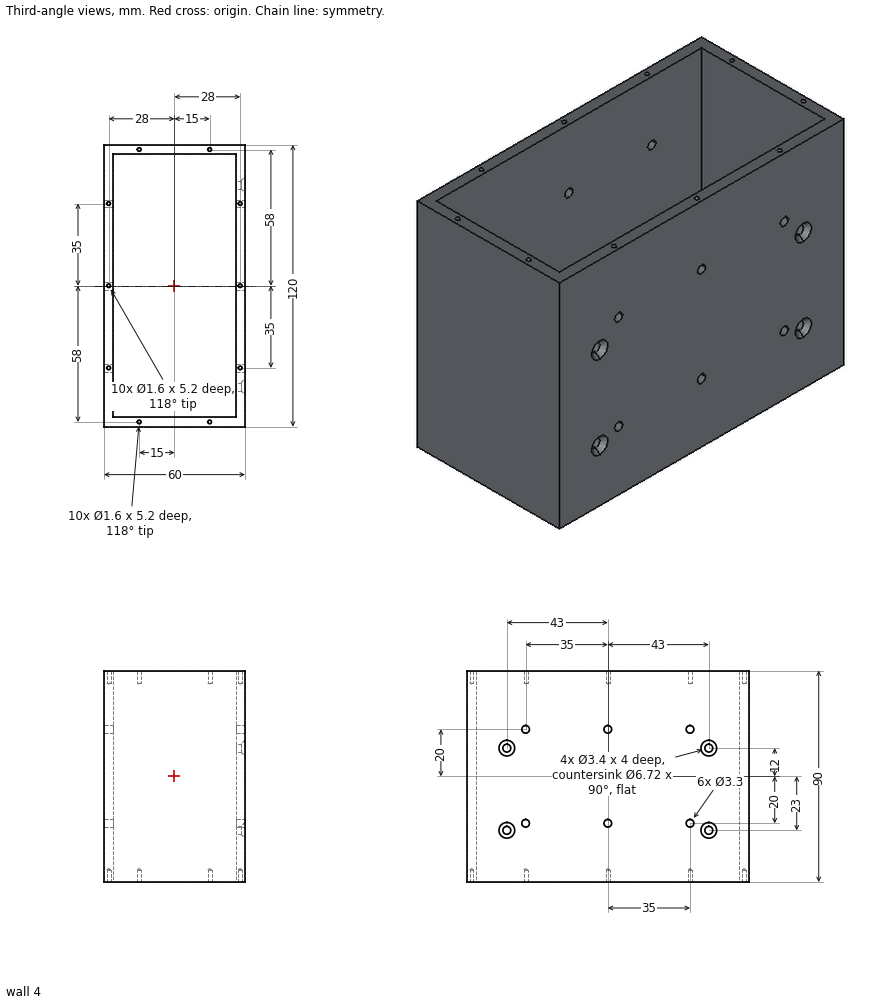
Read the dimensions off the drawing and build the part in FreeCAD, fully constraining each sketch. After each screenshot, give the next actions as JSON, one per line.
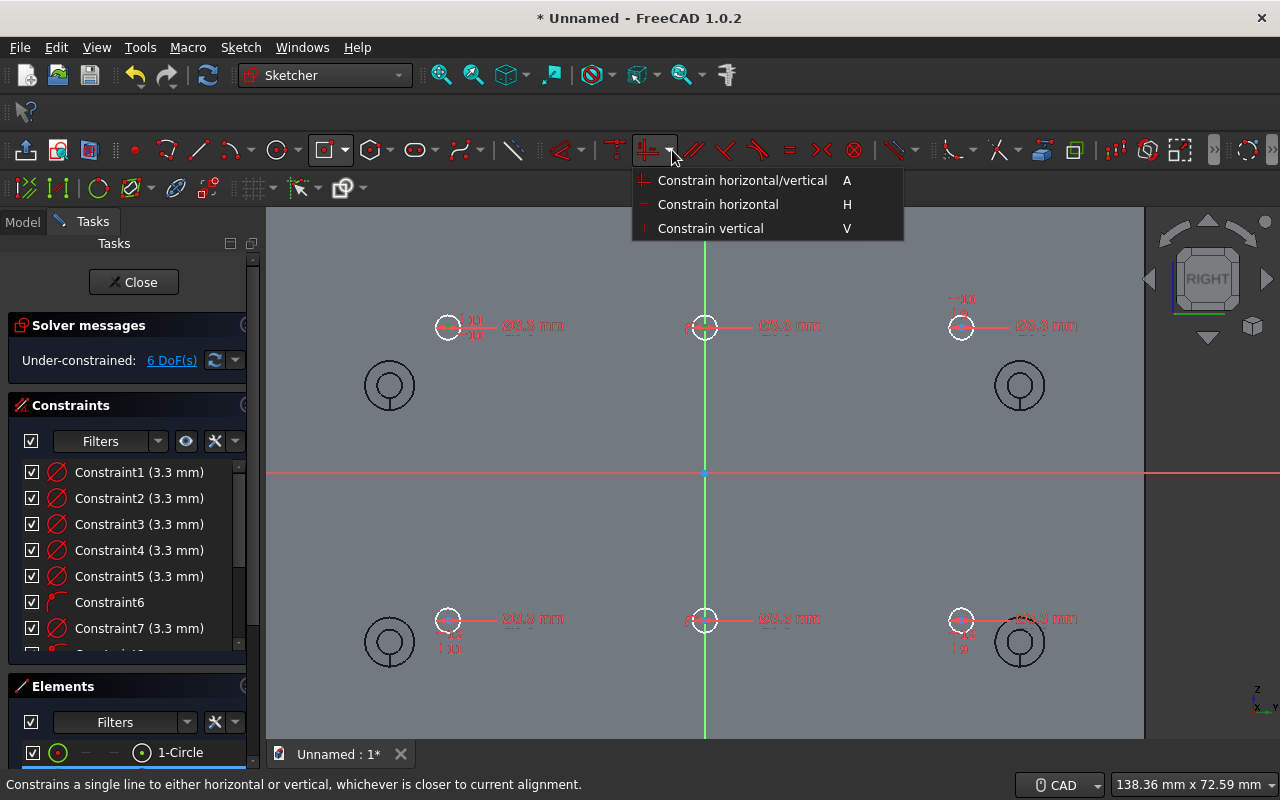
{"action": "left_click", "coordinate": [768, 204]}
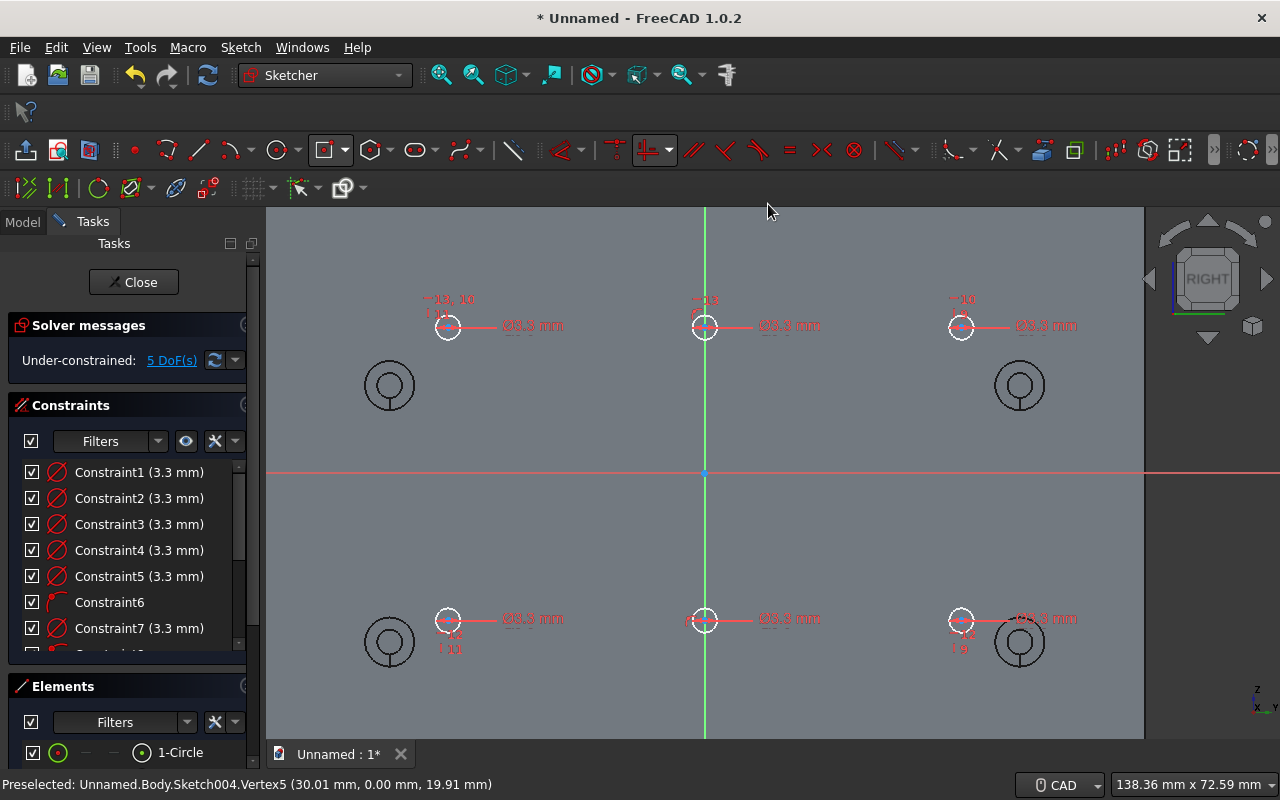
{"action": "left_click", "coordinate": [961, 621]}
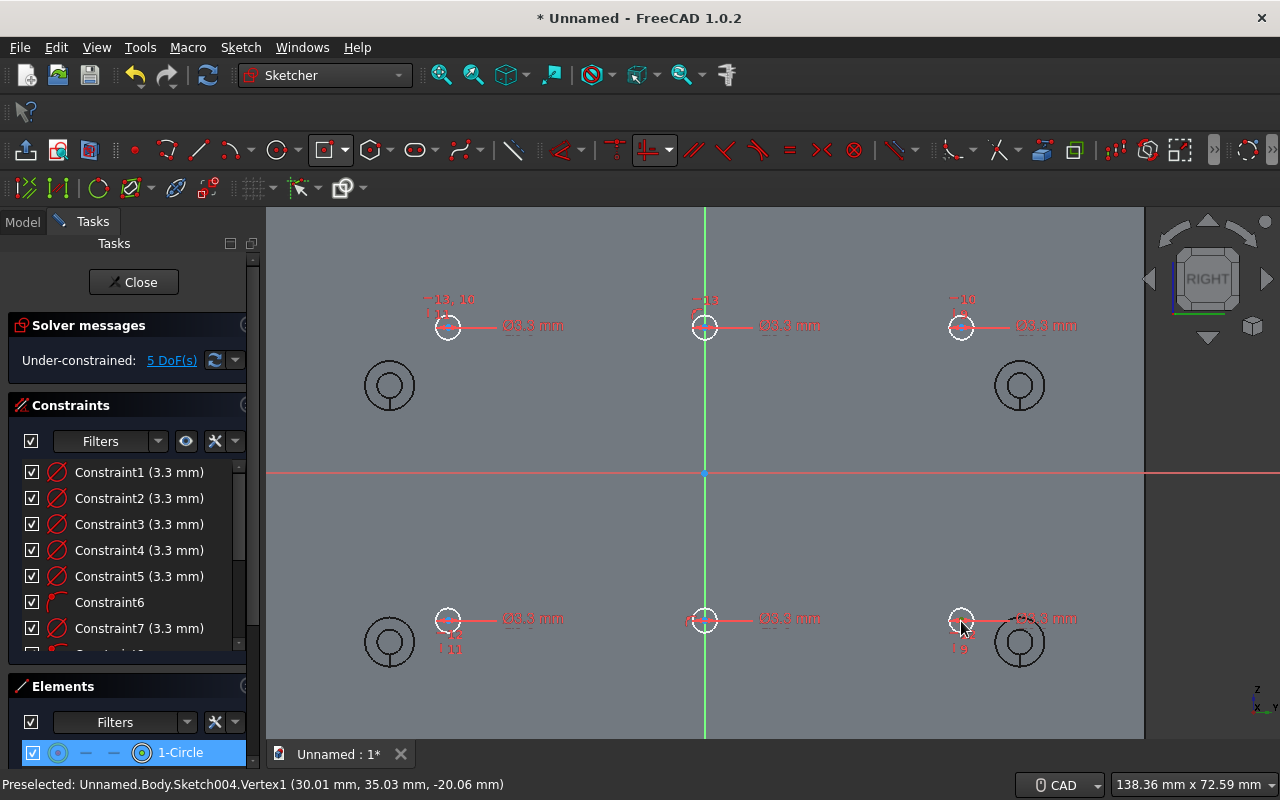
{"action": "left_click", "coordinate": [705, 621]}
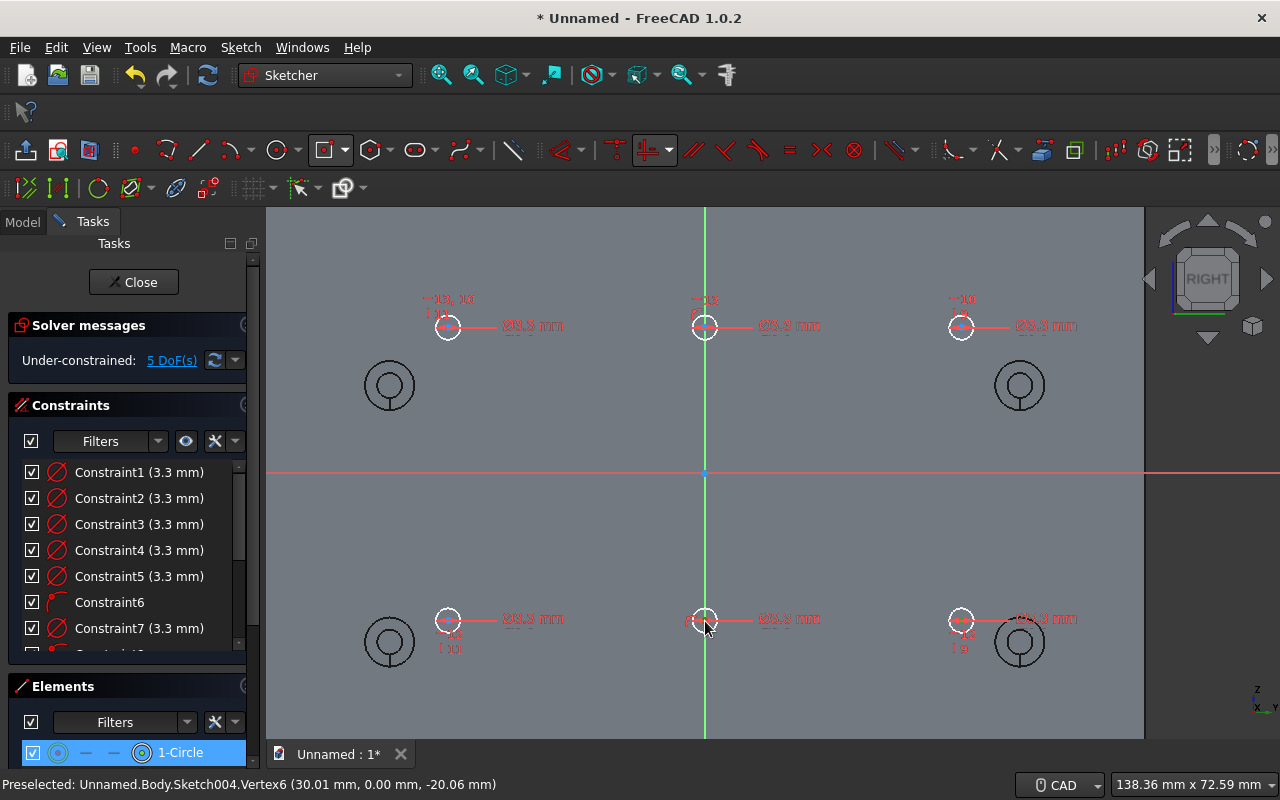
{"action": "left_click", "coordinate": [672, 150]}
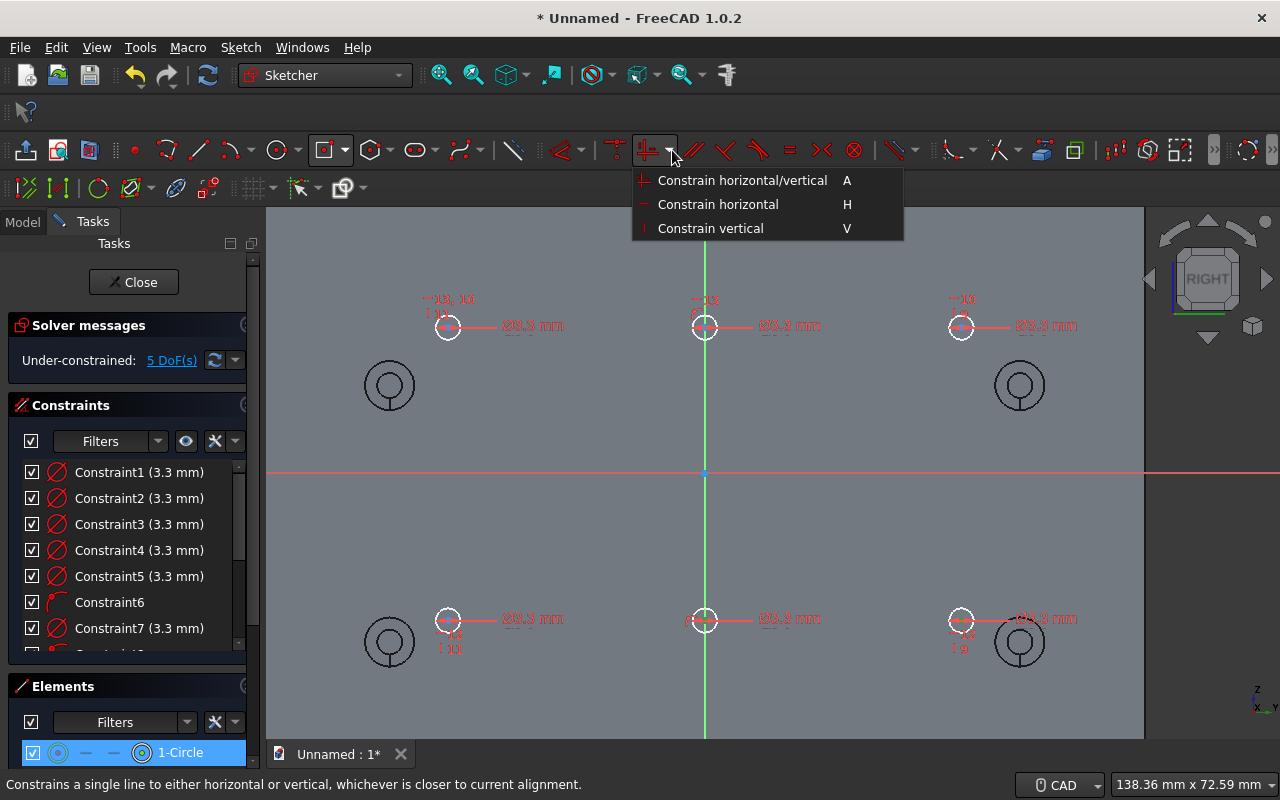
{"action": "left_click", "coordinate": [768, 204]}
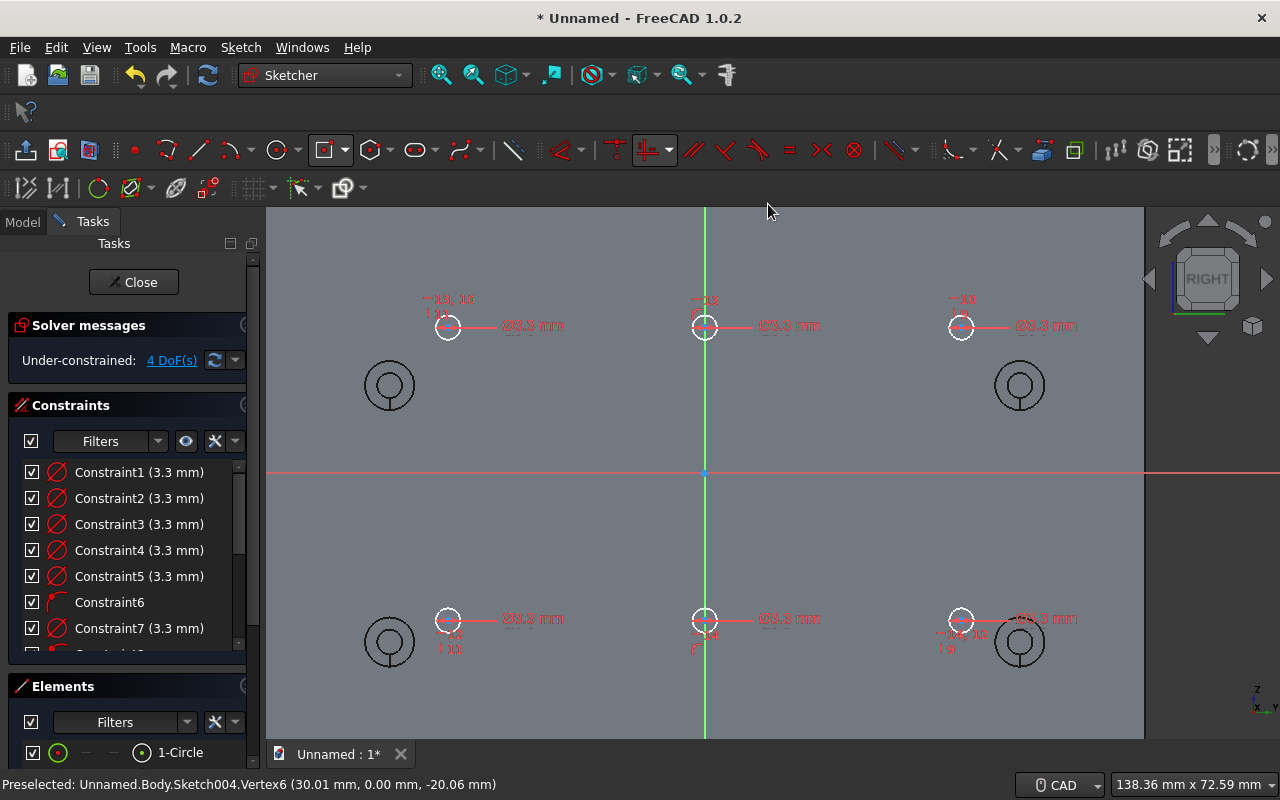
{"action": "left_click", "coordinate": [560, 150]}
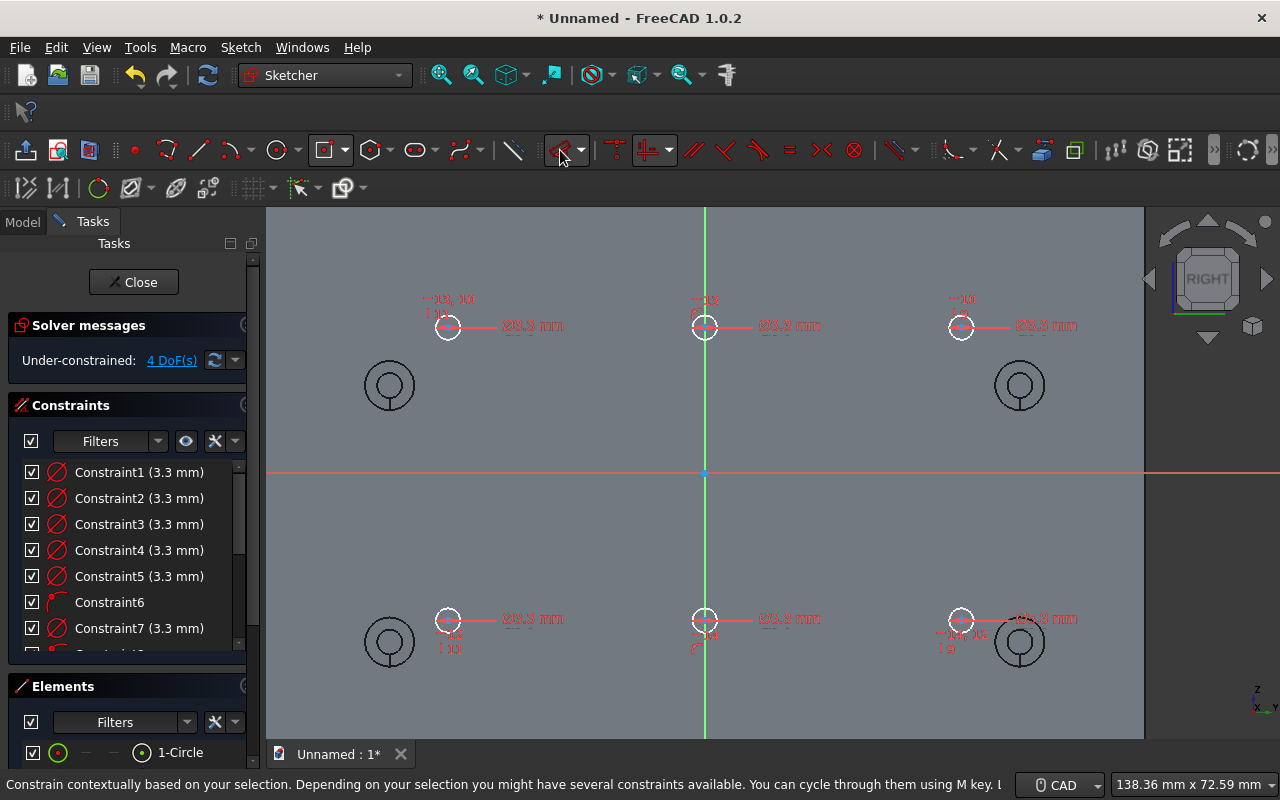
{"action": "left_click", "coordinate": [961, 621]}
{"action": "left_click", "coordinate": [833, 655]}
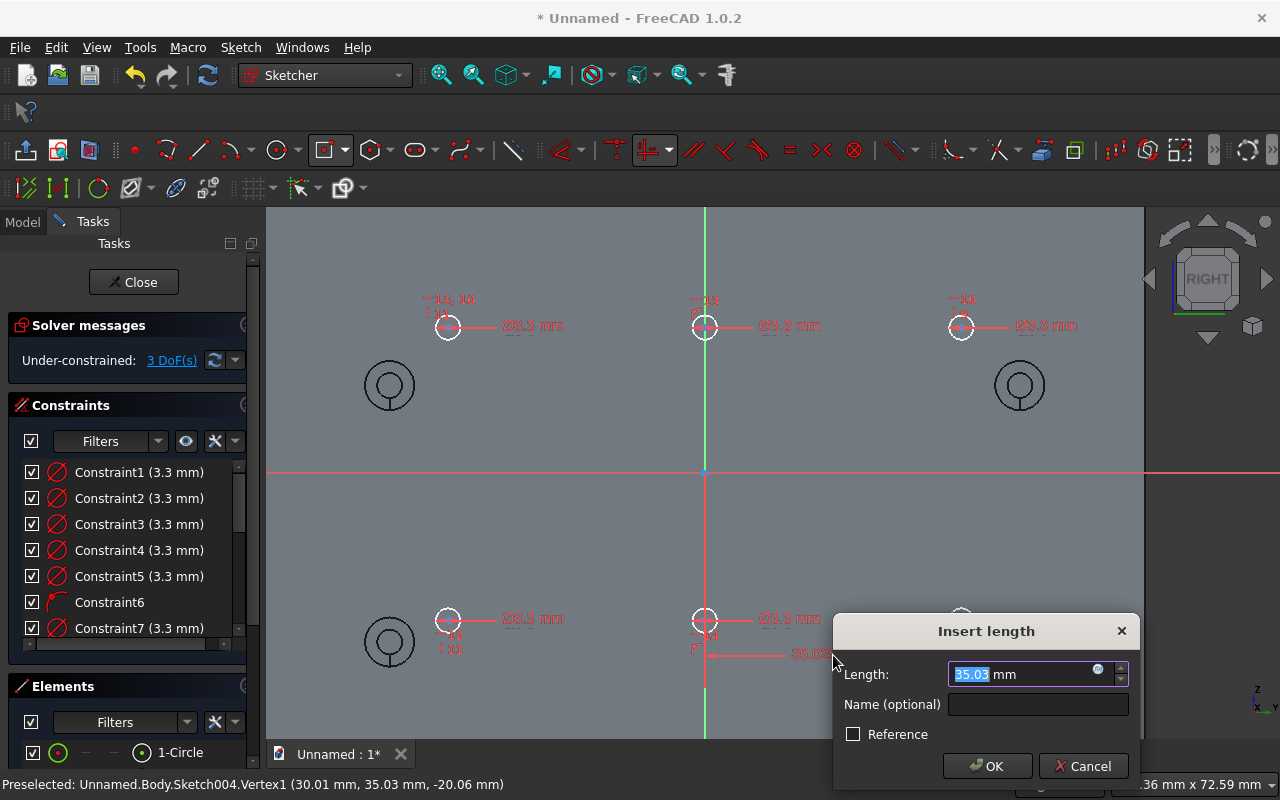
{"action": "type", "text": "35"}
{"action": "key", "text": "Return"}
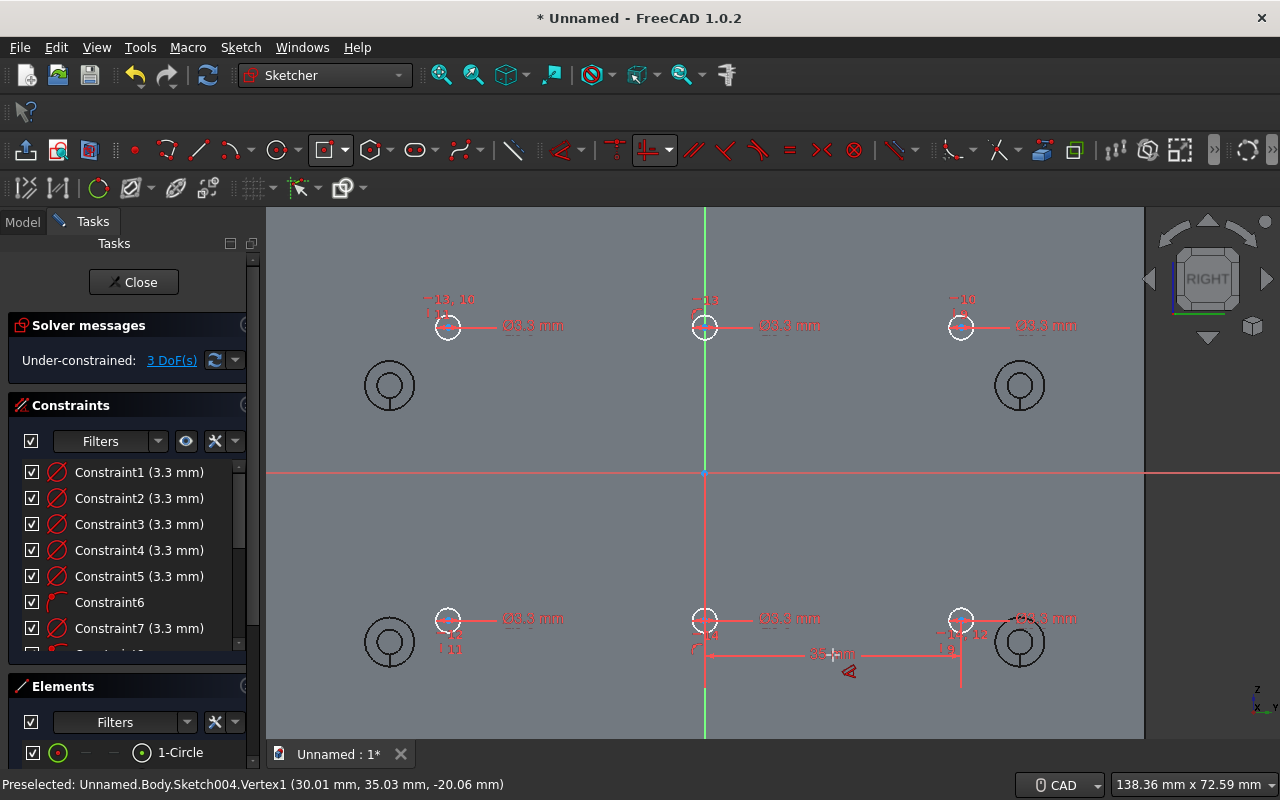
{"action": "left_click", "coordinate": [961, 621]}
{"action": "left_click", "coordinate": [995, 547]}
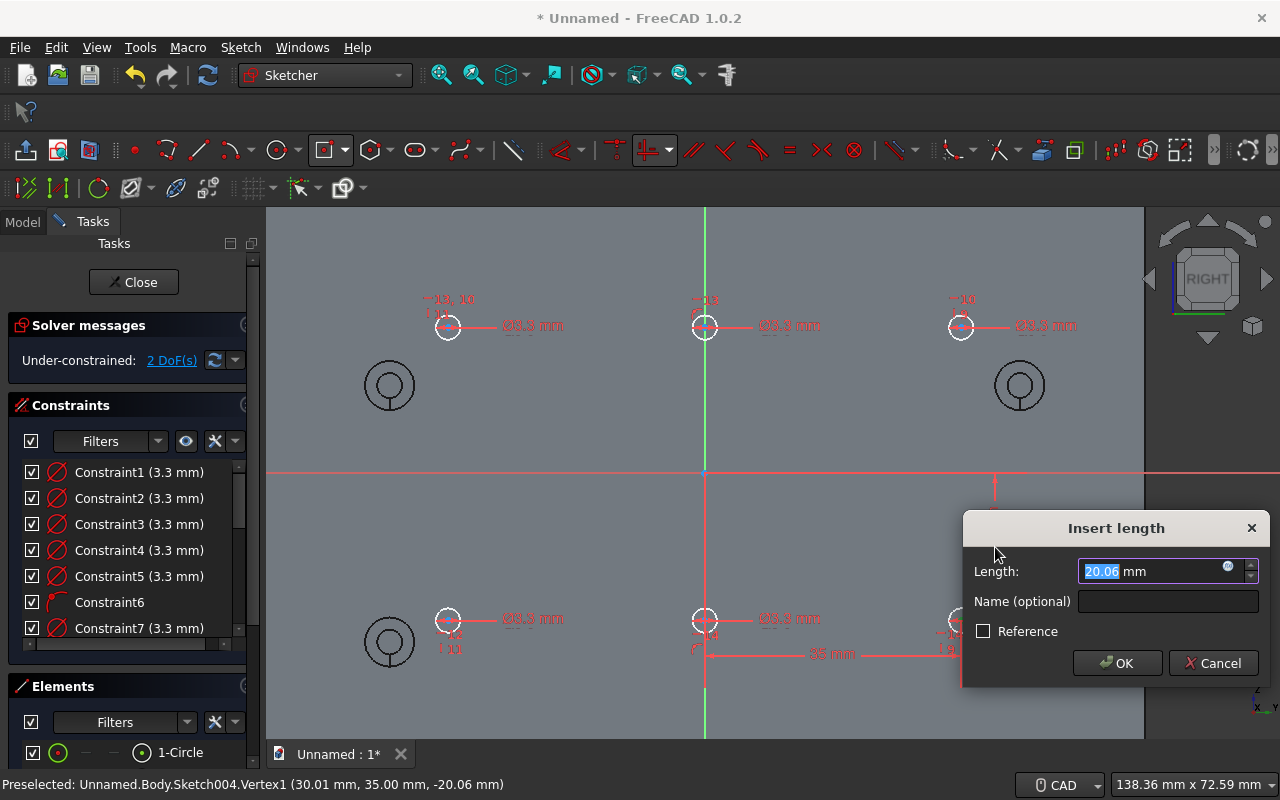
{"action": "type", "text": "20"}
{"action": "key", "text": "Return"}